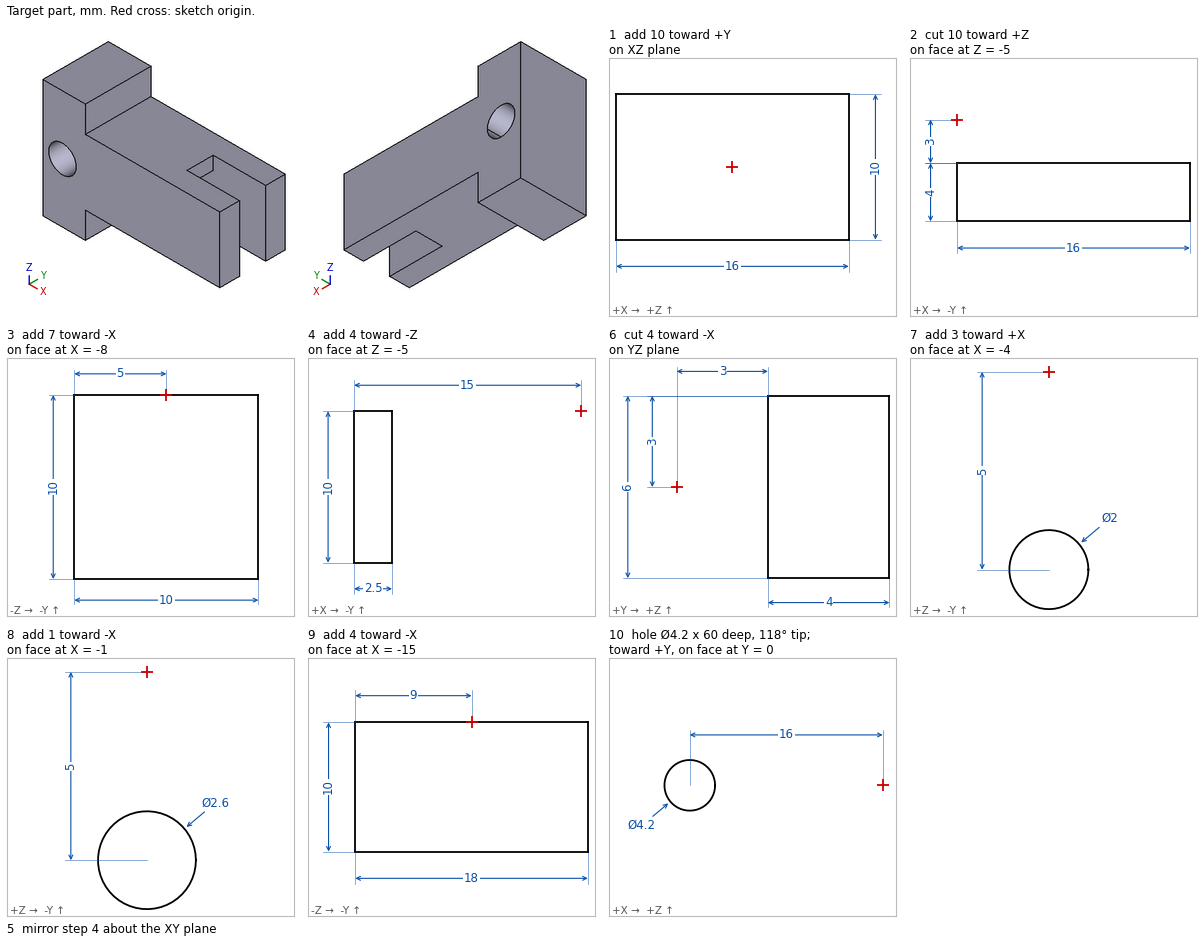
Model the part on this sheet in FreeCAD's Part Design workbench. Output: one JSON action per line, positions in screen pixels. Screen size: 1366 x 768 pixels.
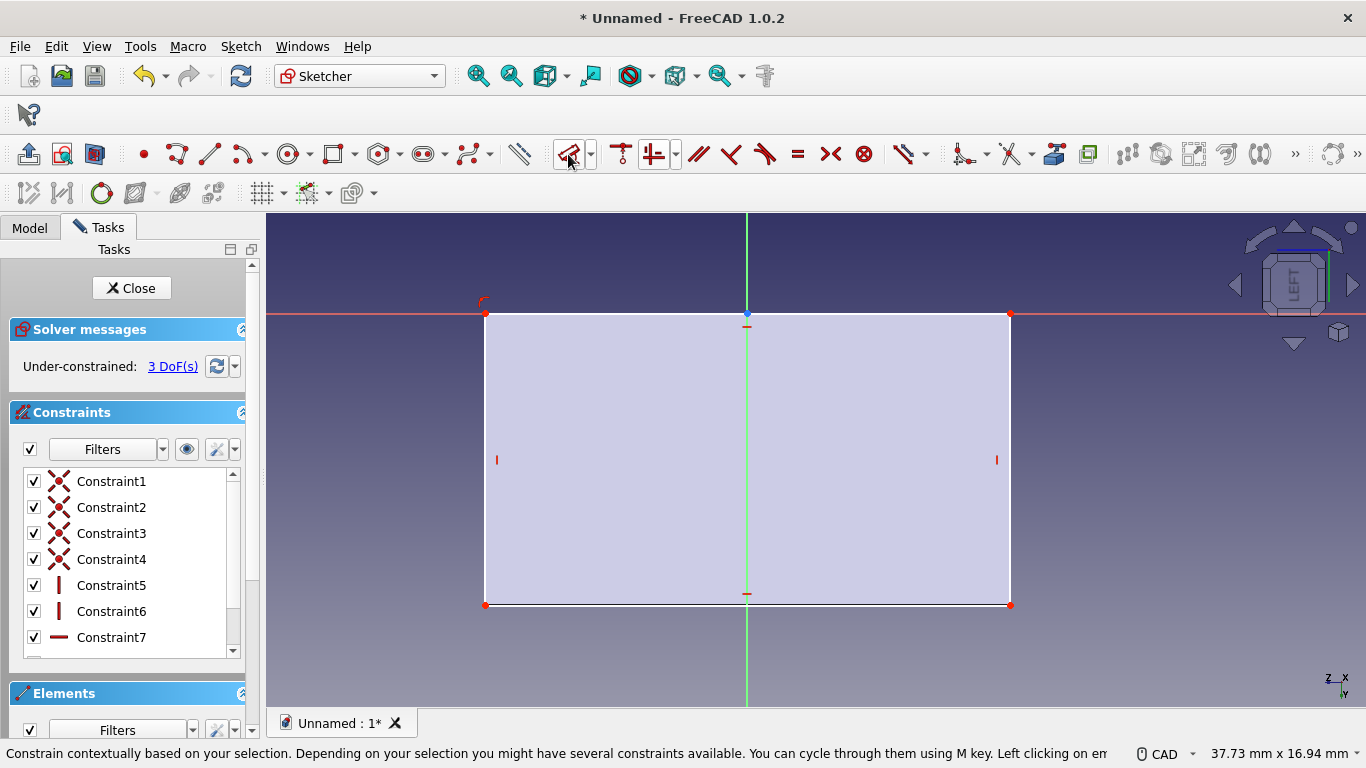
{"action": "left_click", "coordinate": [485, 401]}
{"action": "left_click", "coordinate": [451, 460]}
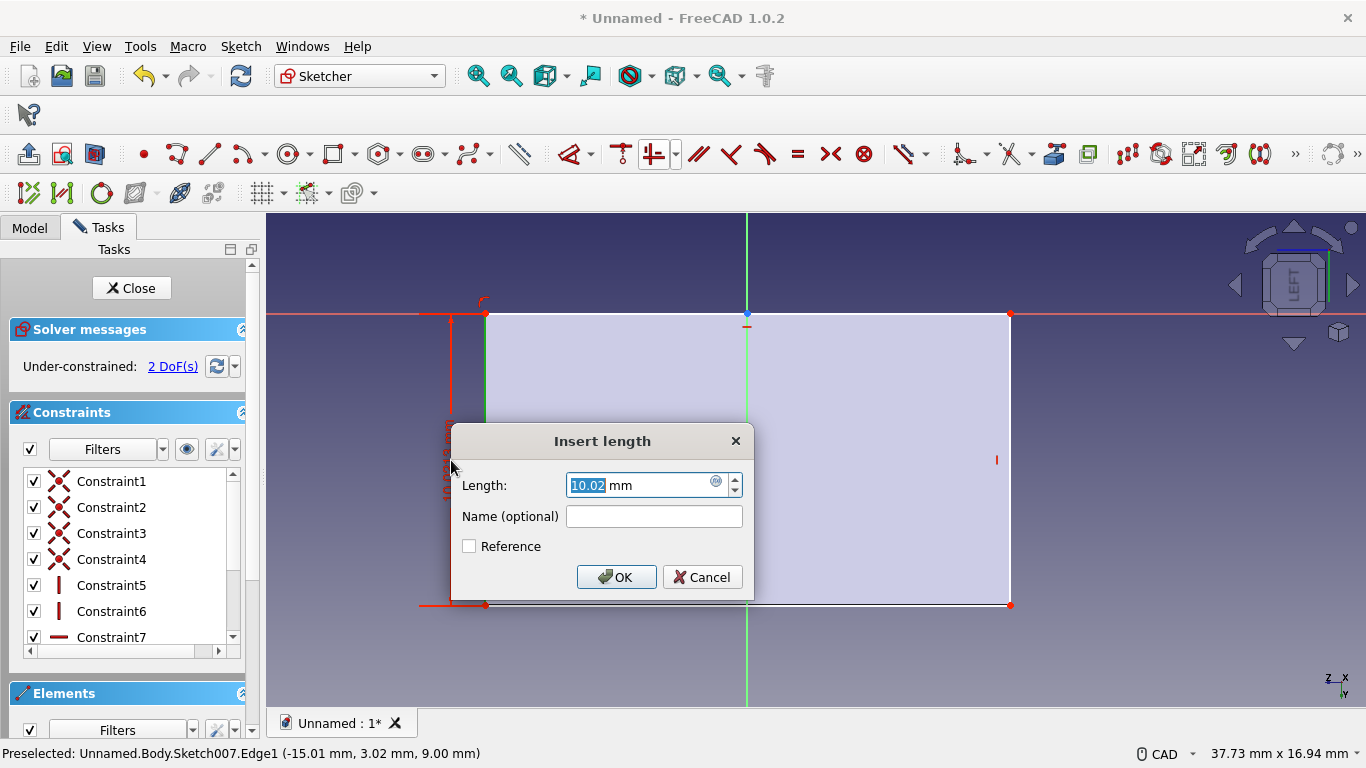
{"action": "type", "text": "10"}
{"action": "key", "text": "Return"}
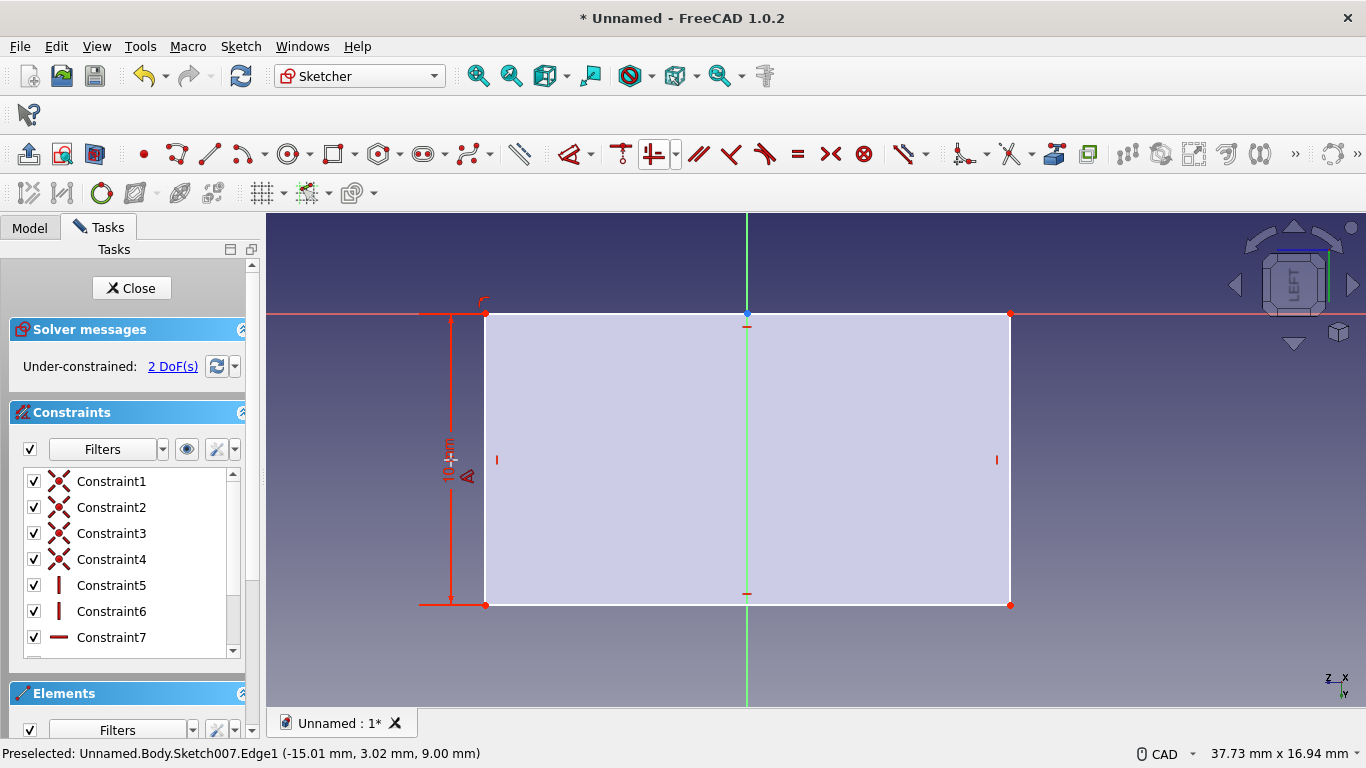
{"action": "left_click", "coordinate": [643, 605]}
{"action": "left_click", "coordinate": [627, 639]}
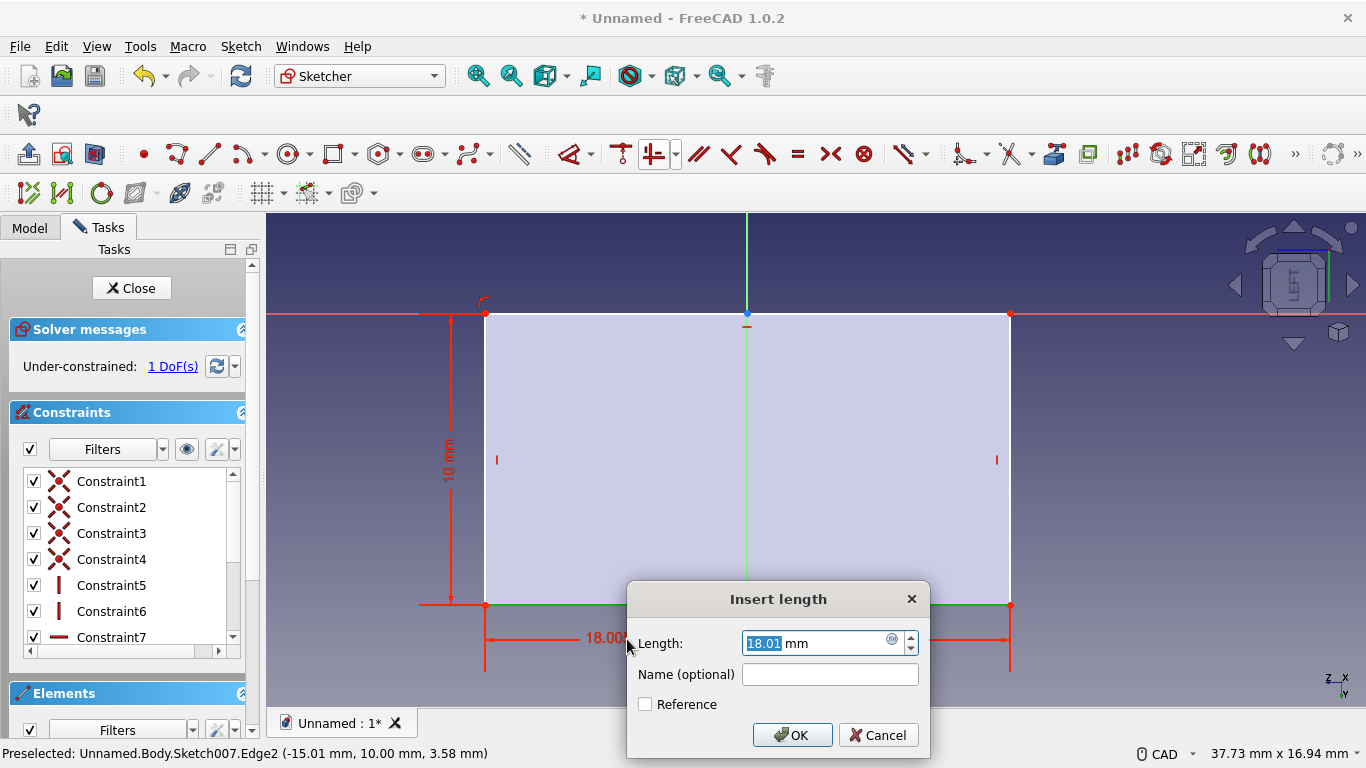
{"action": "type", "text": "18"}
{"action": "key", "text": "Return"}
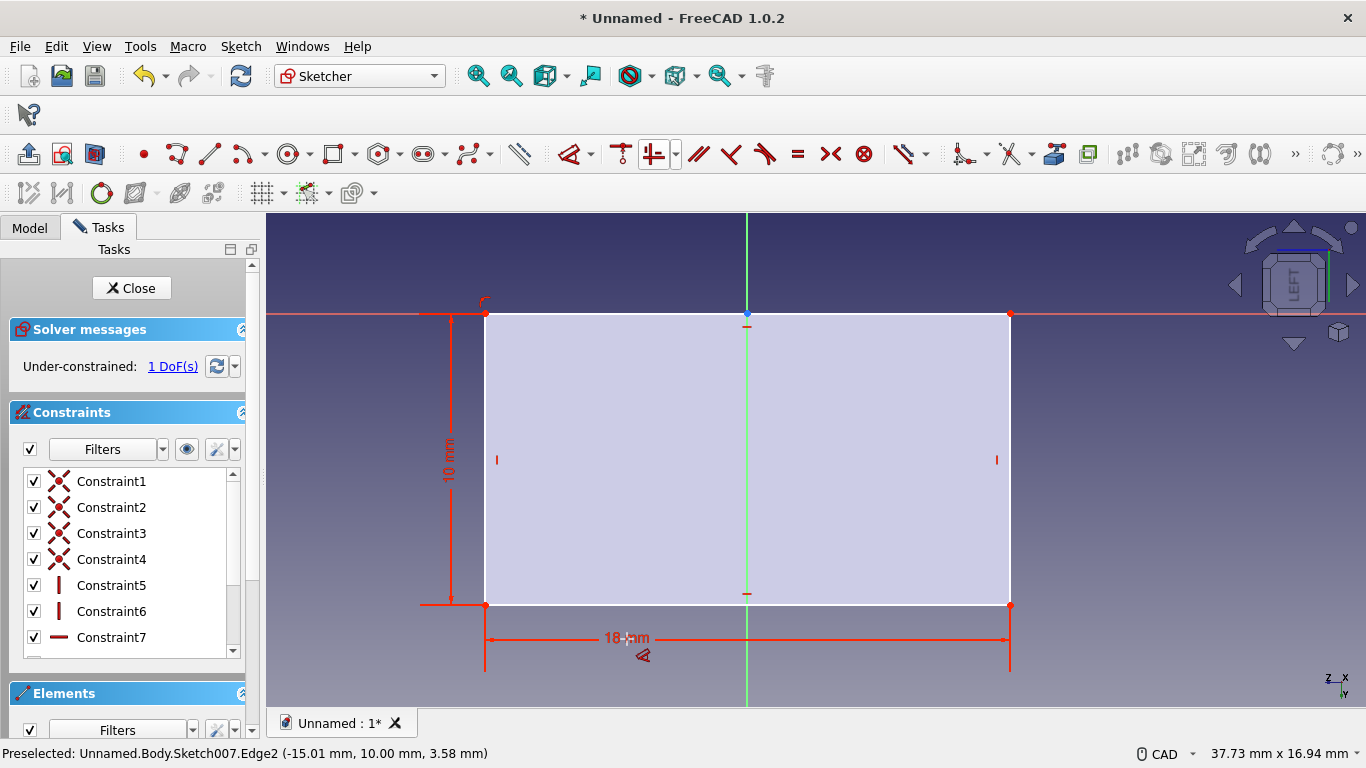
{"action": "left_click", "coordinate": [485, 314]}
{"action": "left_click", "coordinate": [616, 280]}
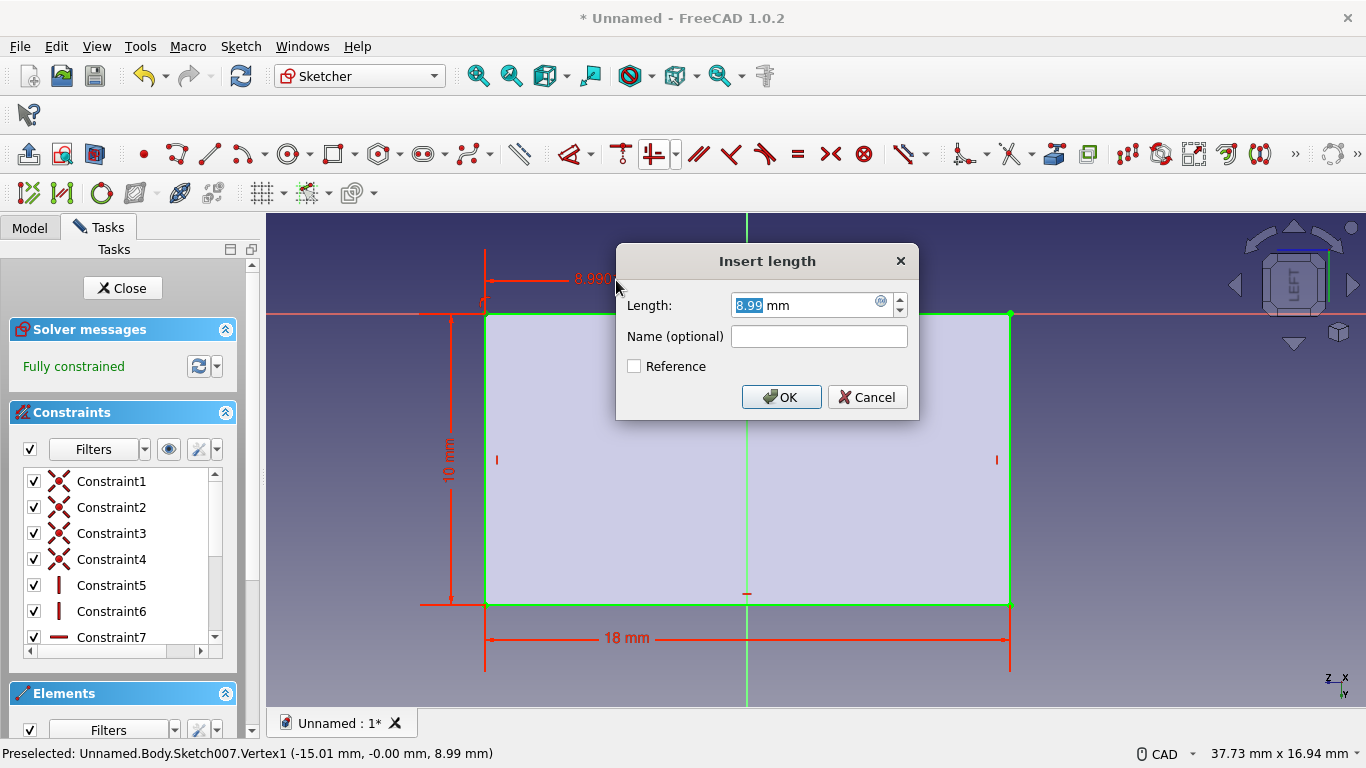
{"action": "type", "text": "9"}
{"action": "key", "text": "Return"}
{"action": "key", "text": "Escape"}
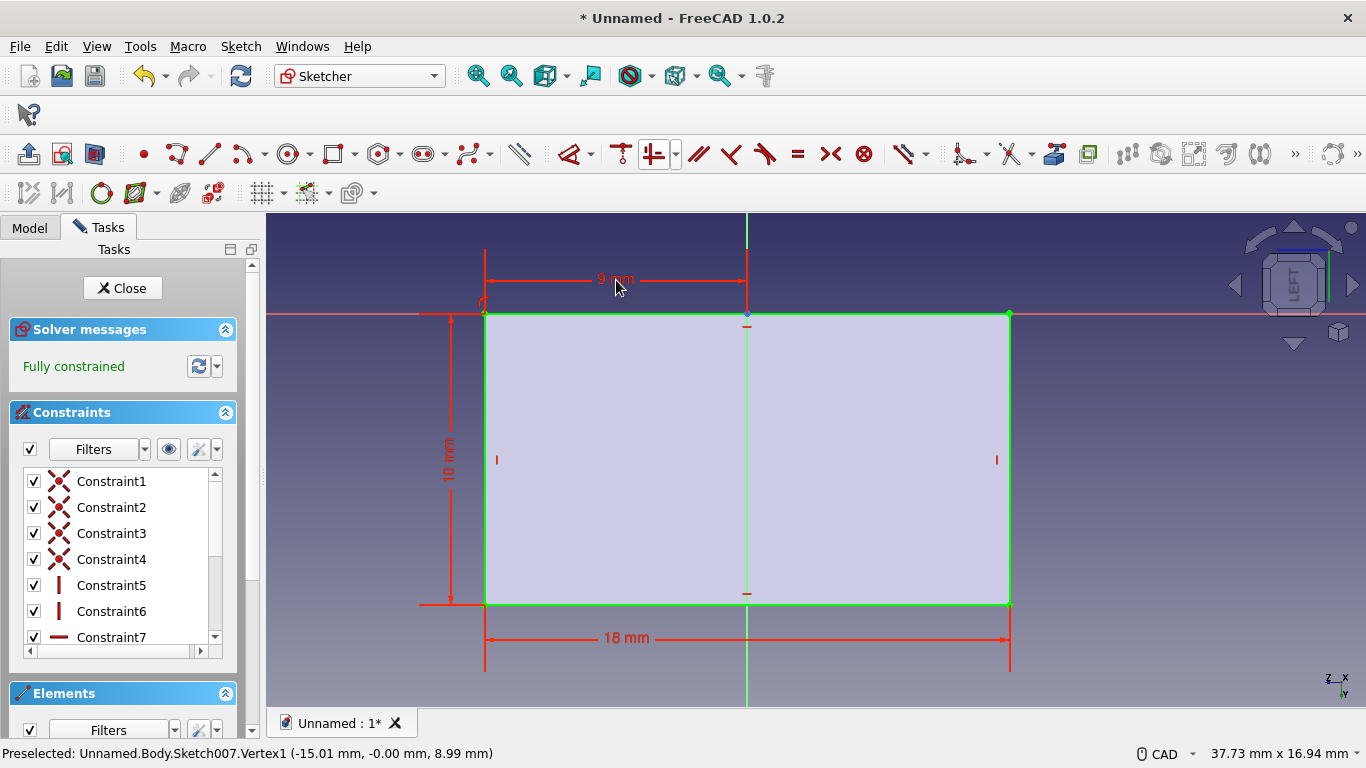
{"action": "left_click", "coordinate": [123, 288]}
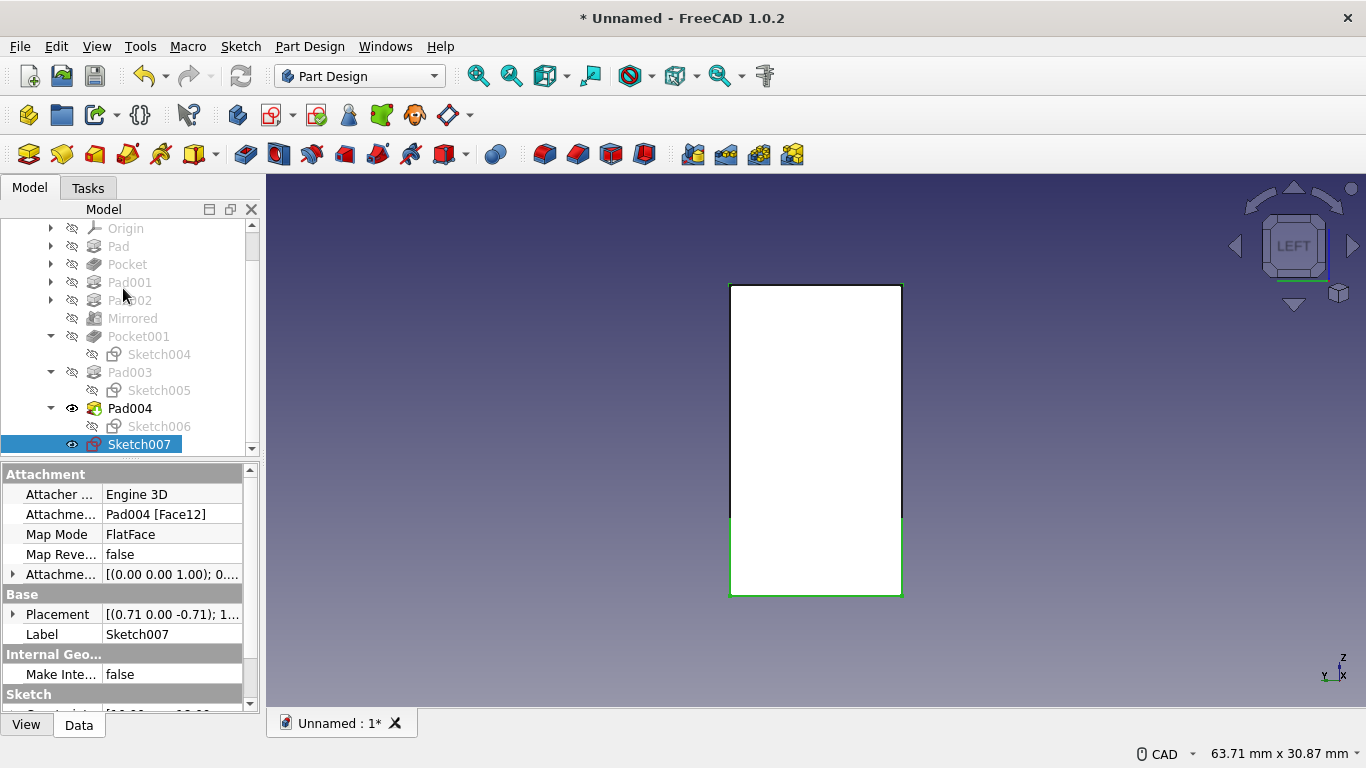
{"action": "left_click", "coordinate": [29, 154]}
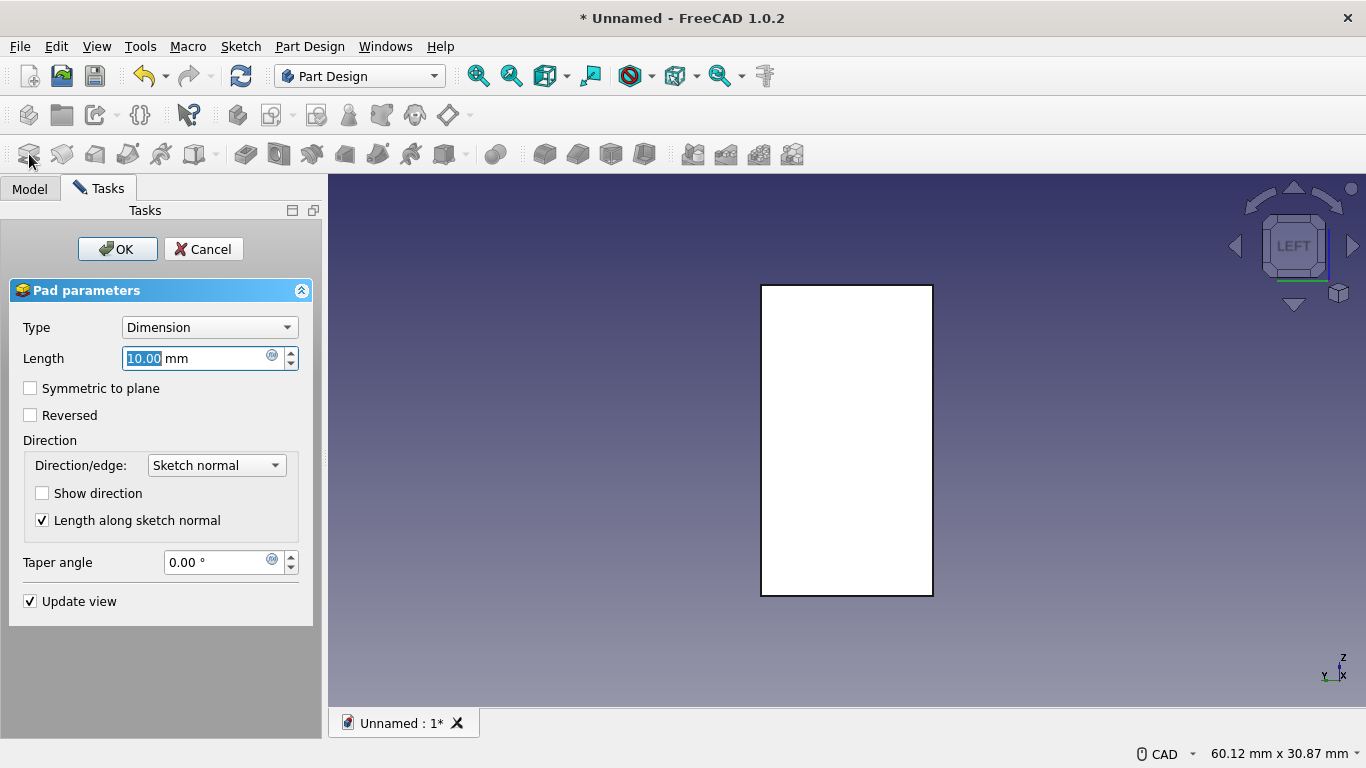
{"action": "type", "text": "4"}
{"action": "key", "text": "Tab"}